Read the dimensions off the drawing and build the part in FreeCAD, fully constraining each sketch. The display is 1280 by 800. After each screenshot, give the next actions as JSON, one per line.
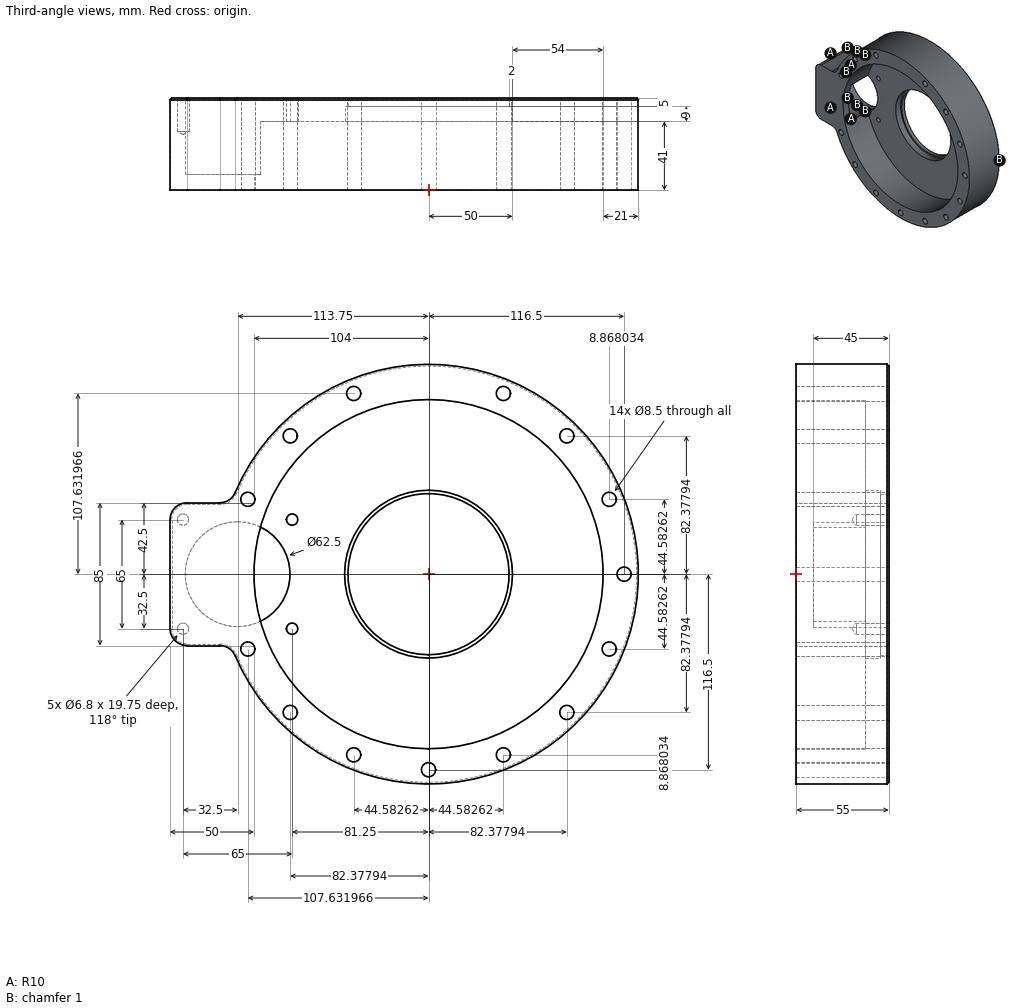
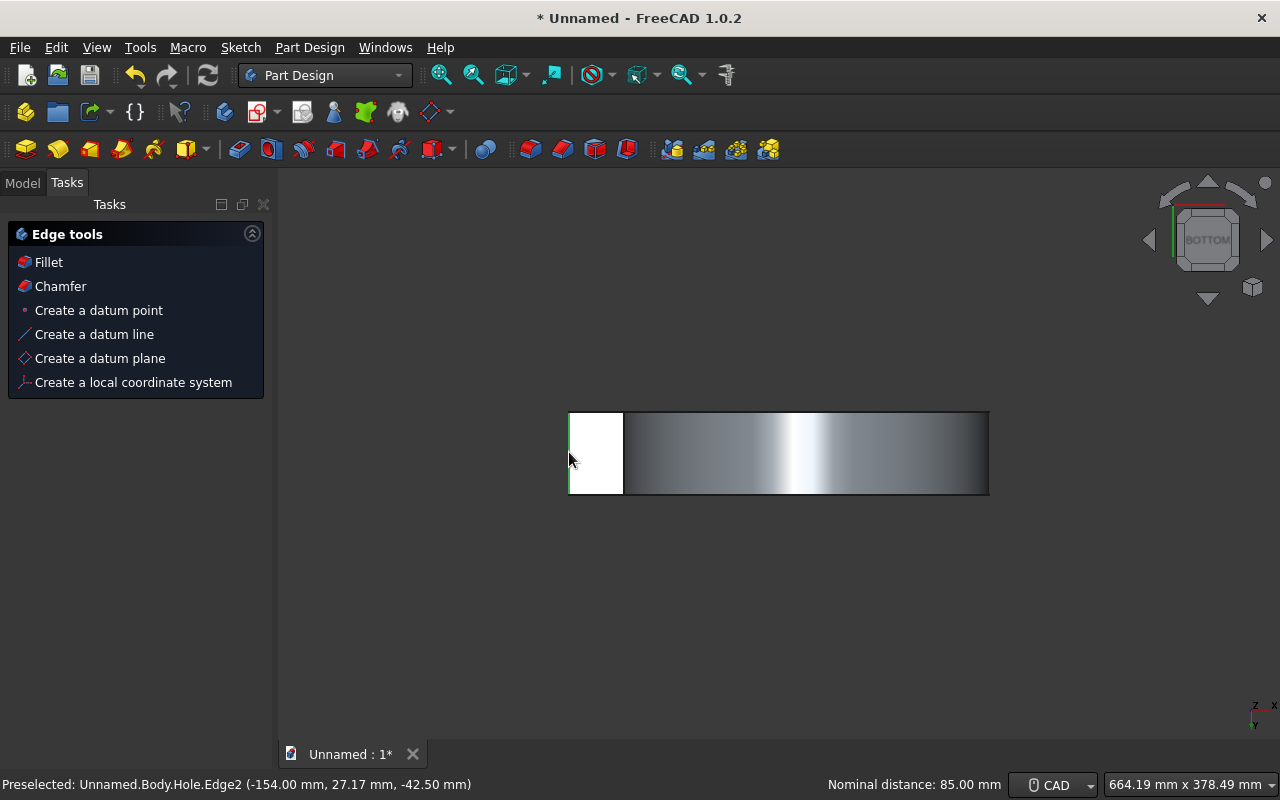
{"action": "key", "text": "4"}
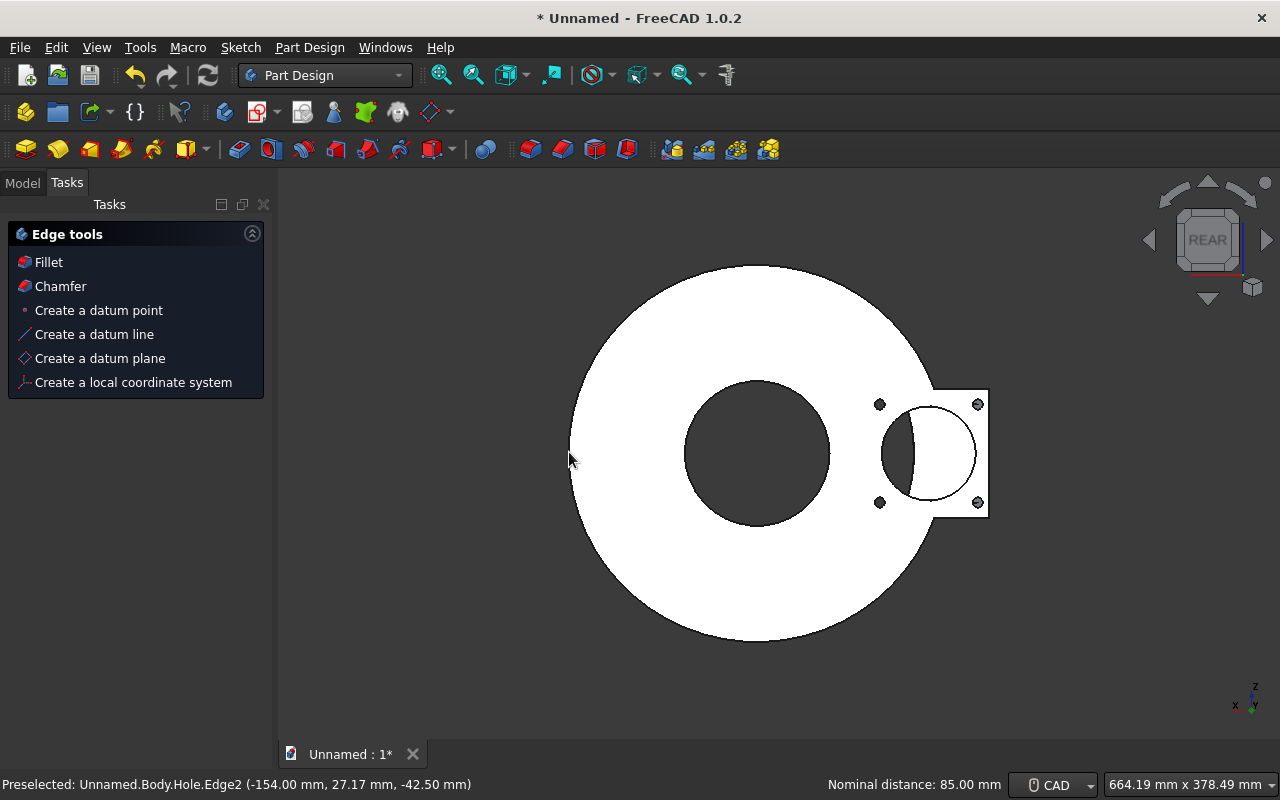
{"action": "key", "text": "6"}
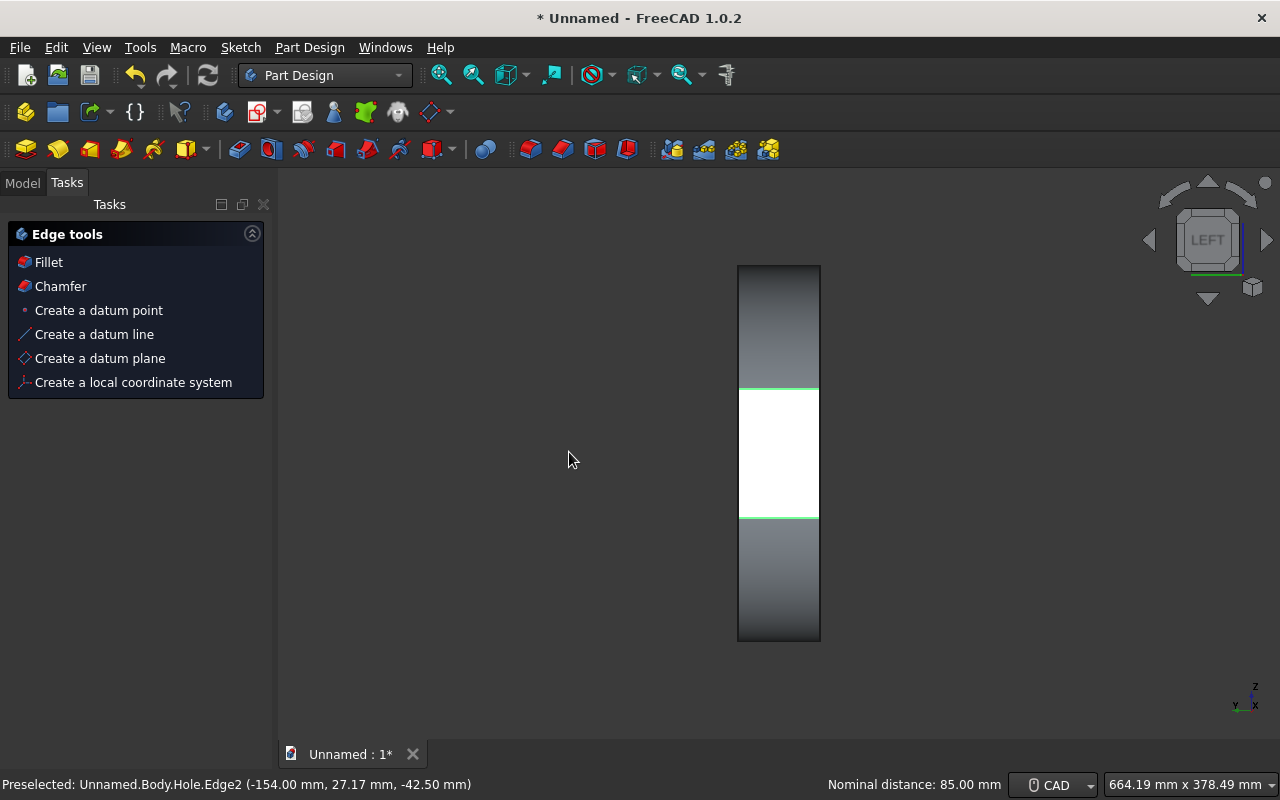
{"action": "key", "text": "v 3"}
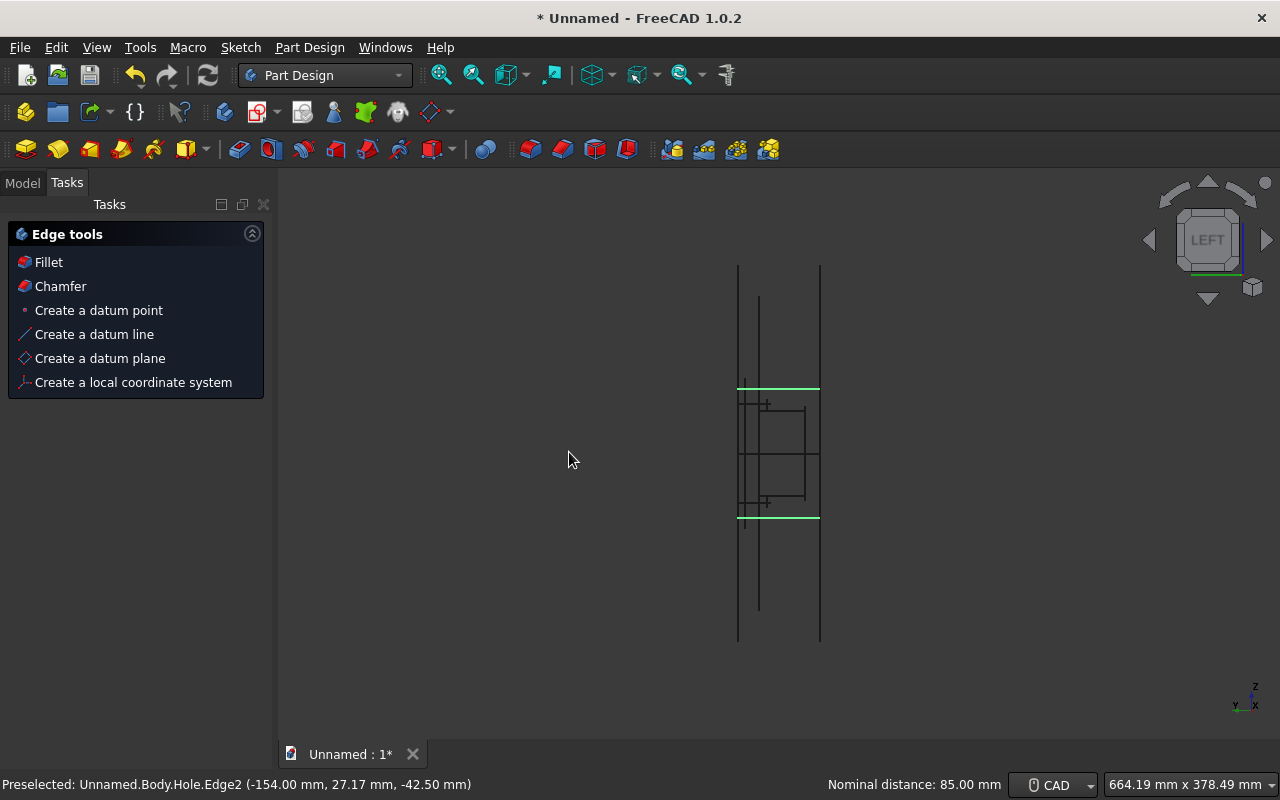
{"action": "key", "text": "0"}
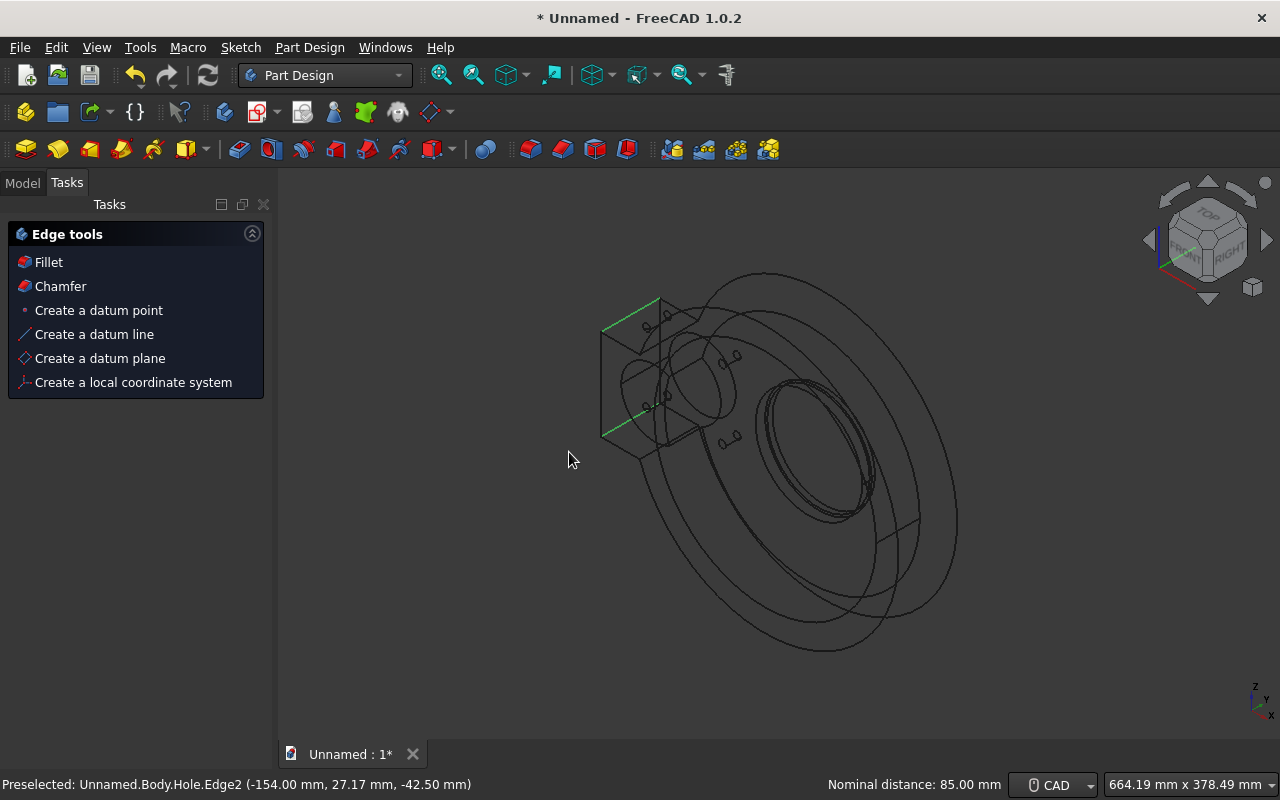
{"action": "left_click", "coordinate": [669, 337], "text": "ctrl"}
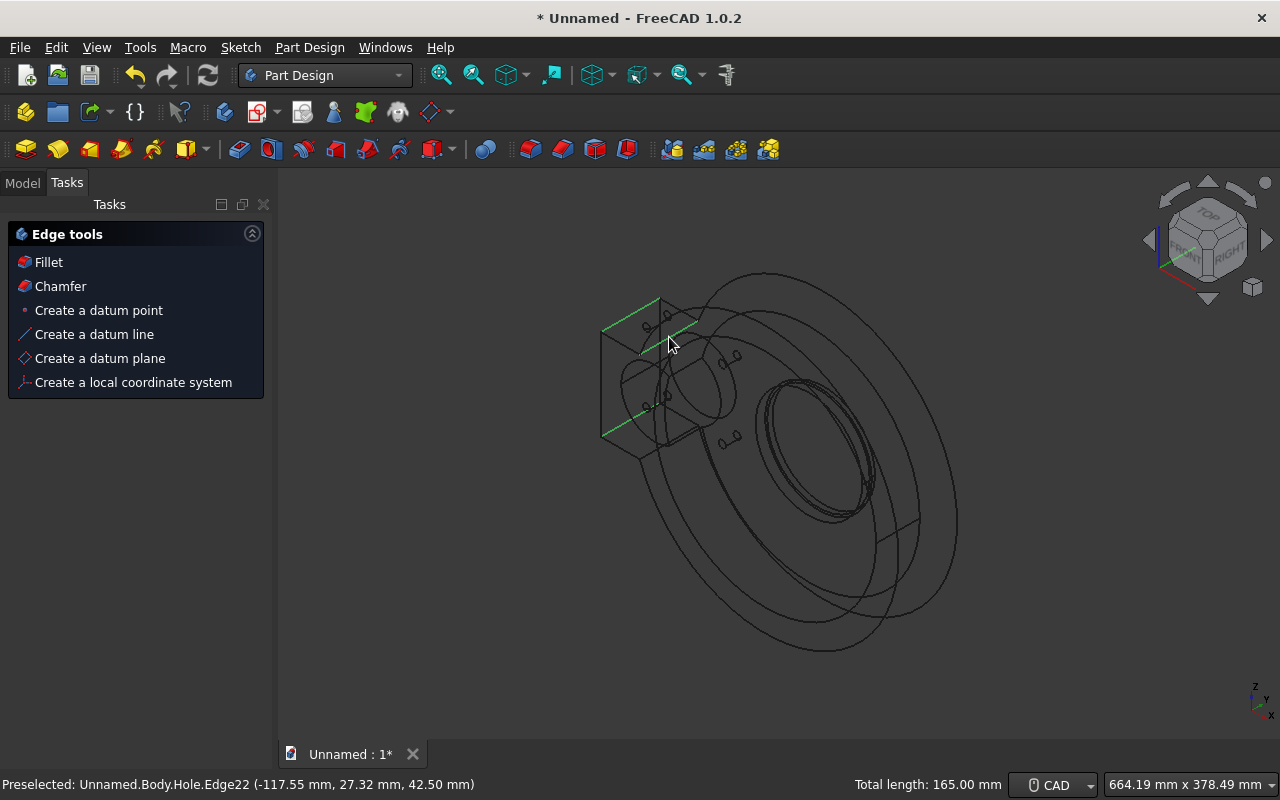
{"action": "left_click", "coordinate": [651, 452], "text": "ctrl"}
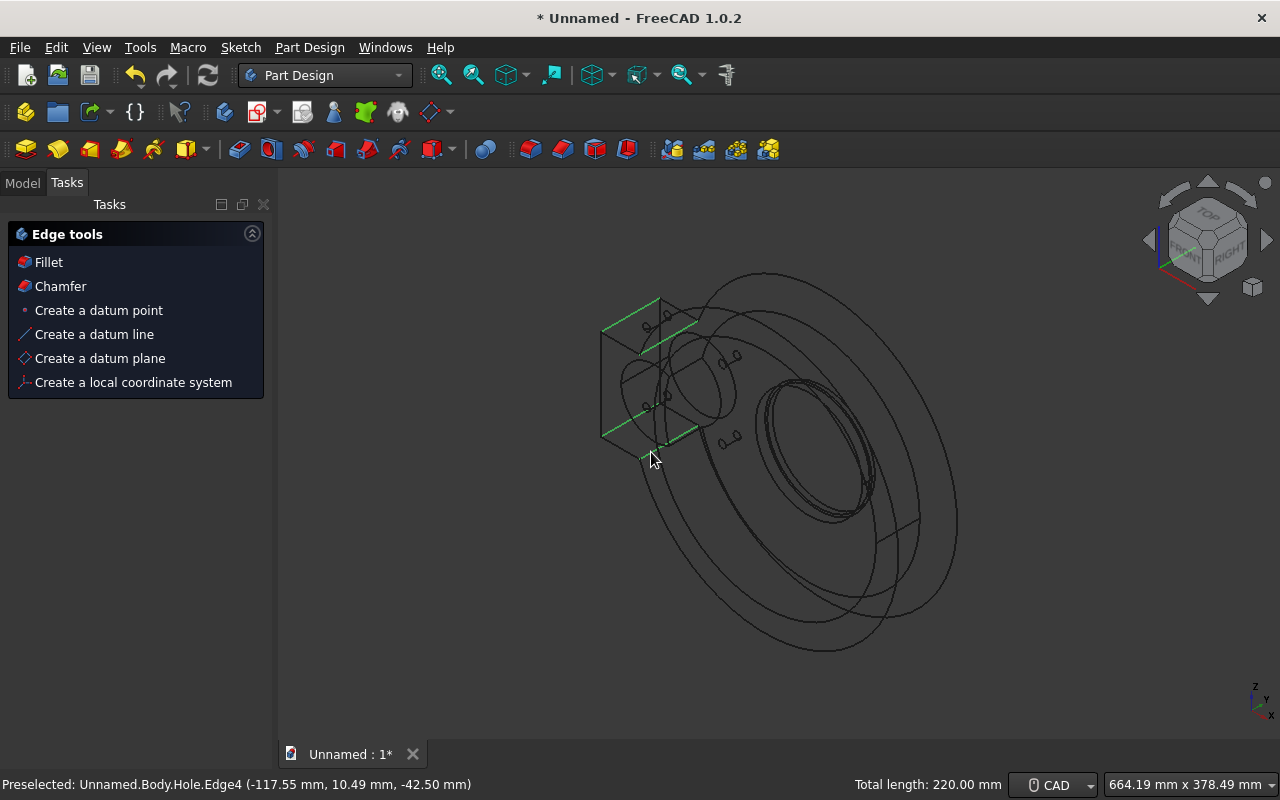
{"action": "key", "text": "v 1"}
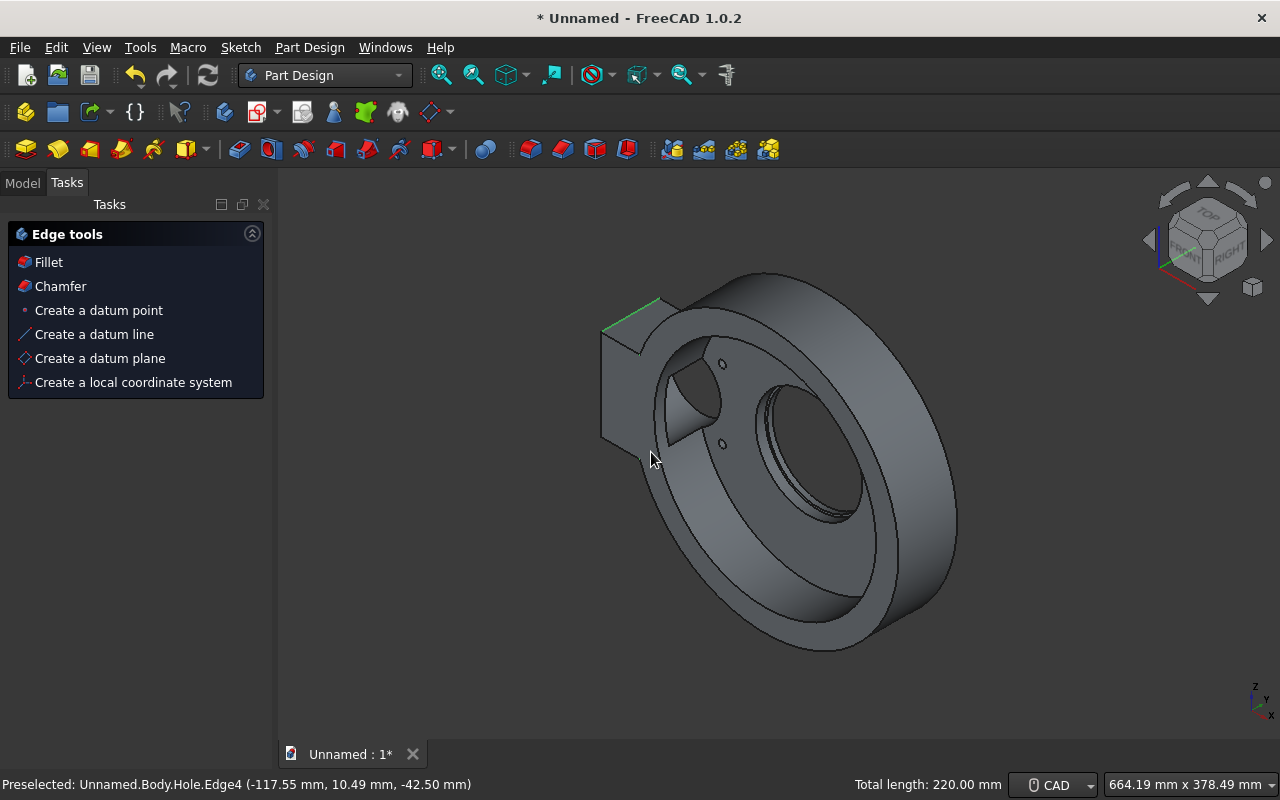
{"action": "left_click", "coordinate": [532, 150]}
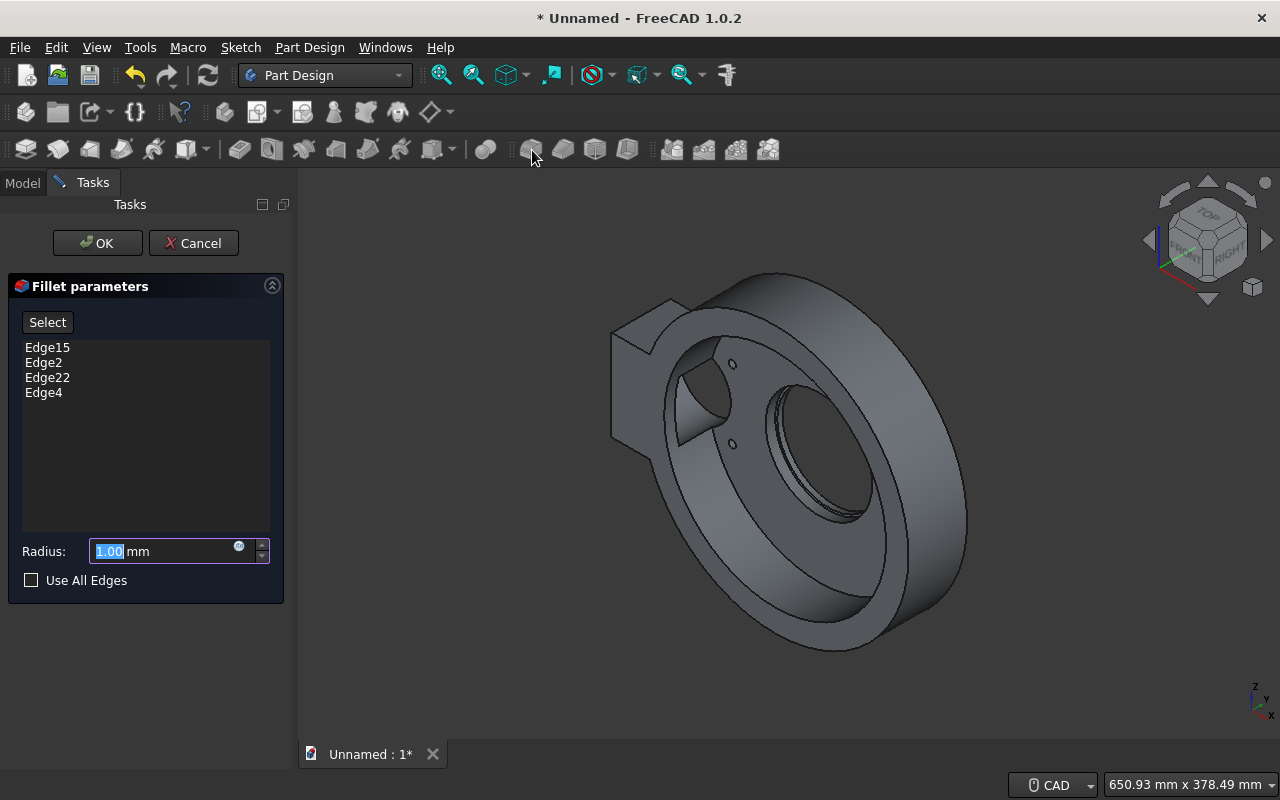
{"action": "type", "text": "10"}
{"action": "key", "text": "Tab"}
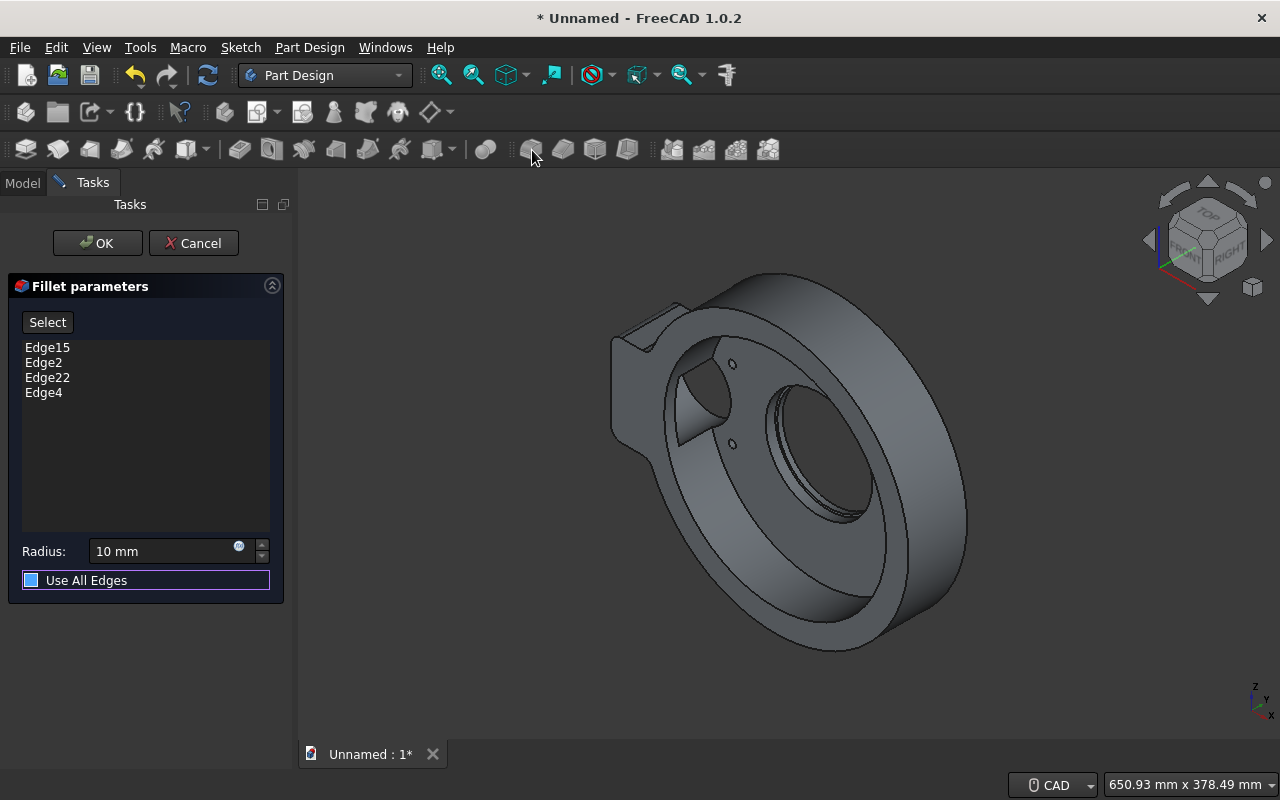
{"action": "left_click", "coordinate": [98, 243]}